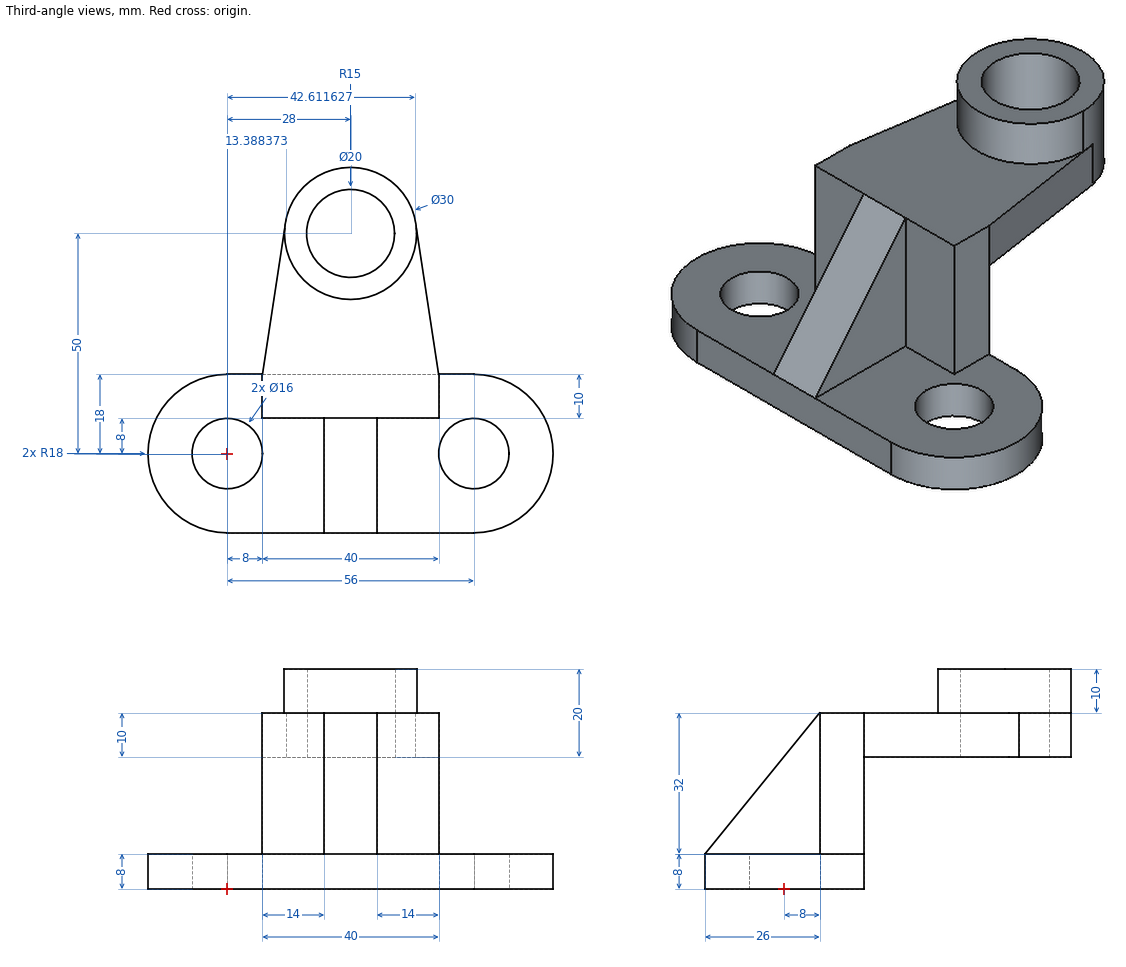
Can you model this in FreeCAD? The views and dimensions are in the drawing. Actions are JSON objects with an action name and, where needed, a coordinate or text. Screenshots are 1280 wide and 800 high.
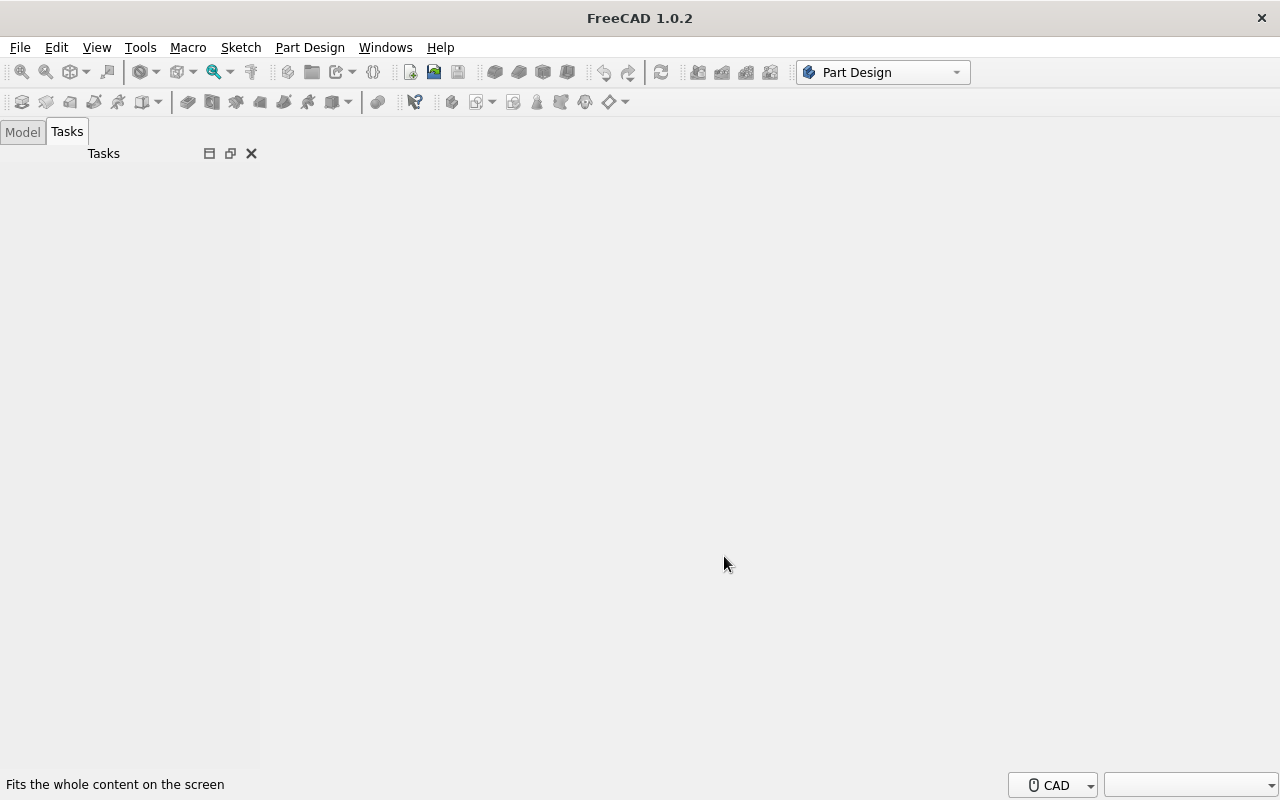
{"action": "left_click", "coordinate": [410, 72]}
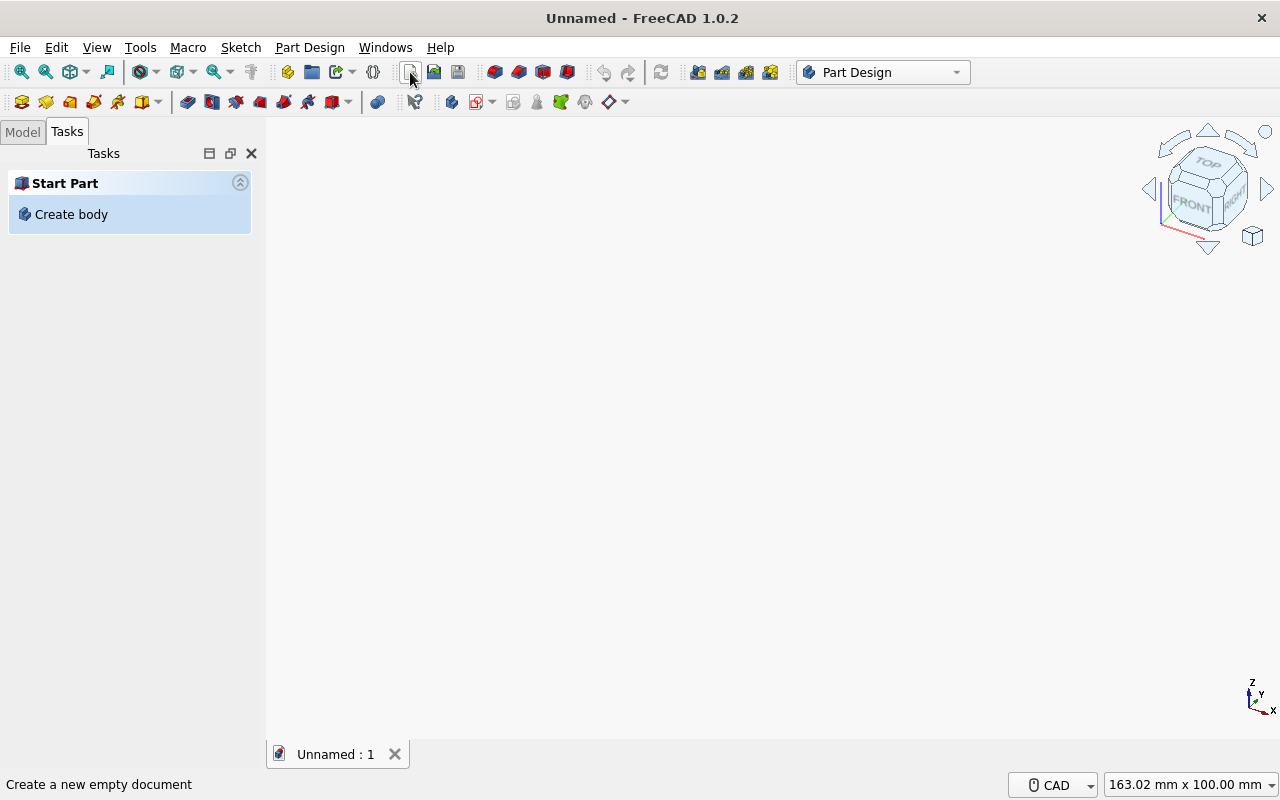
{"action": "left_click", "coordinate": [476, 102]}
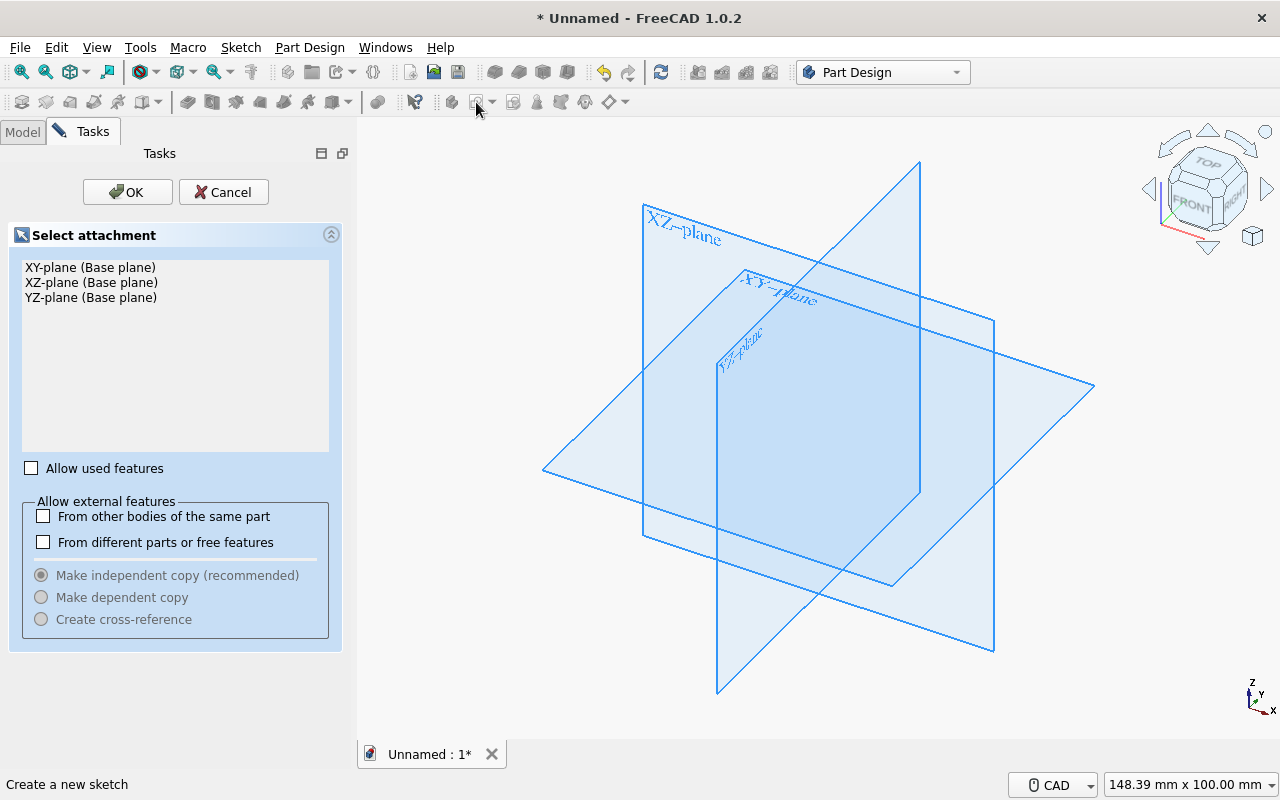
{"action": "left_click", "coordinate": [82, 268]}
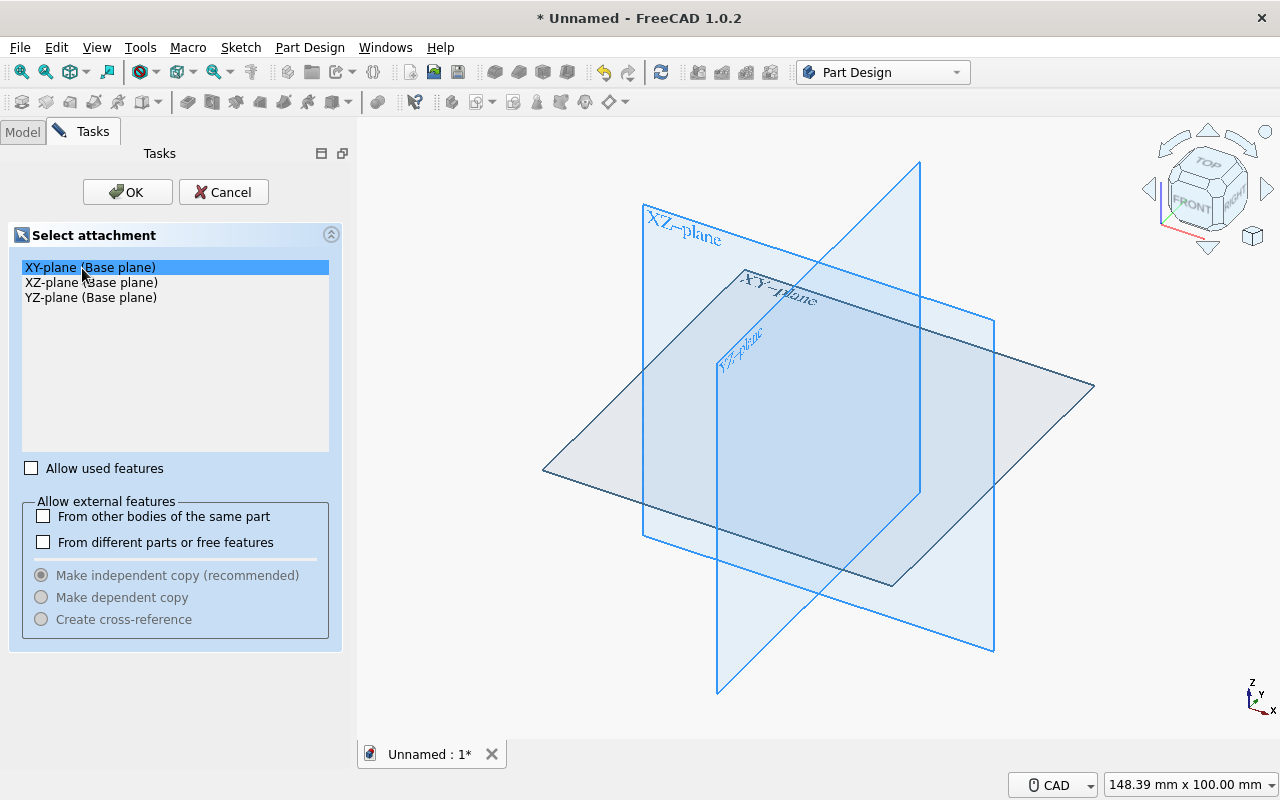
{"action": "left_click", "coordinate": [128, 192]}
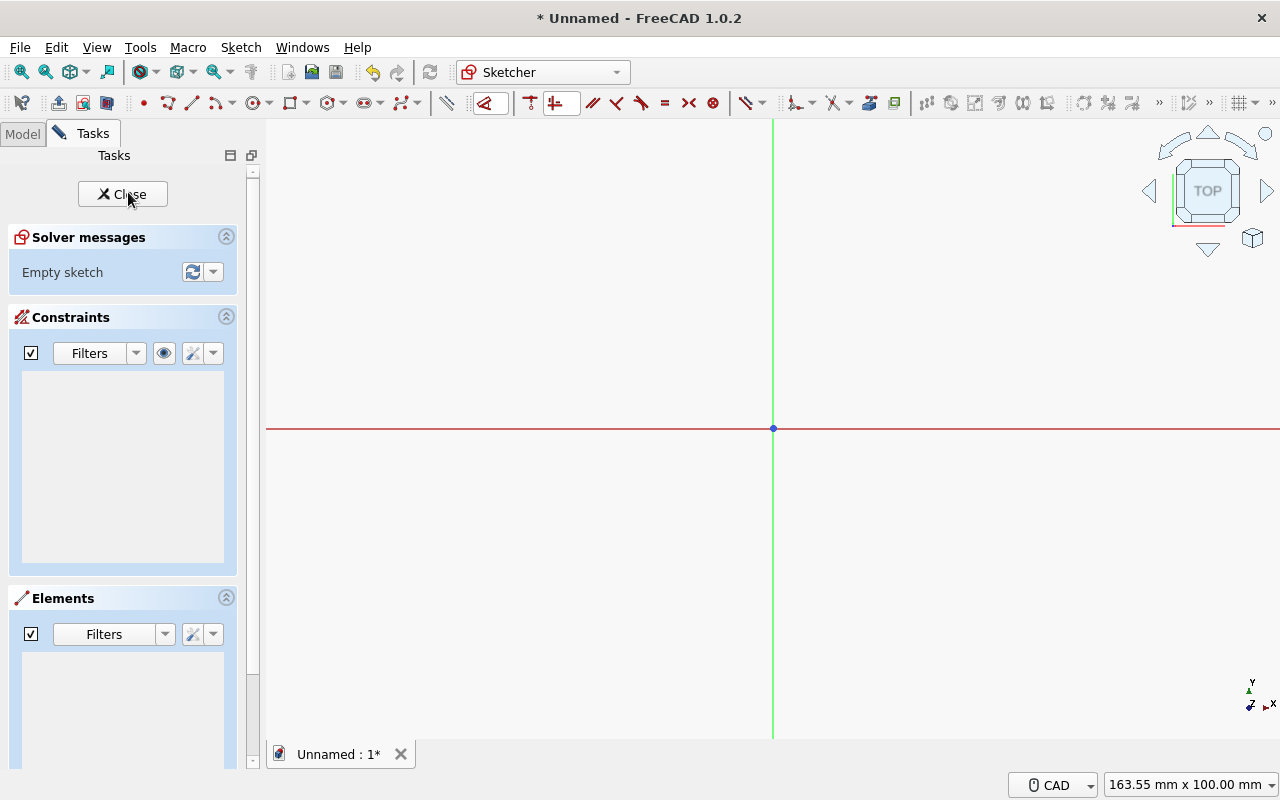
{"action": "scroll", "coordinate": [294, 429], "scroll_direction": "down", "scroll_amount": 1}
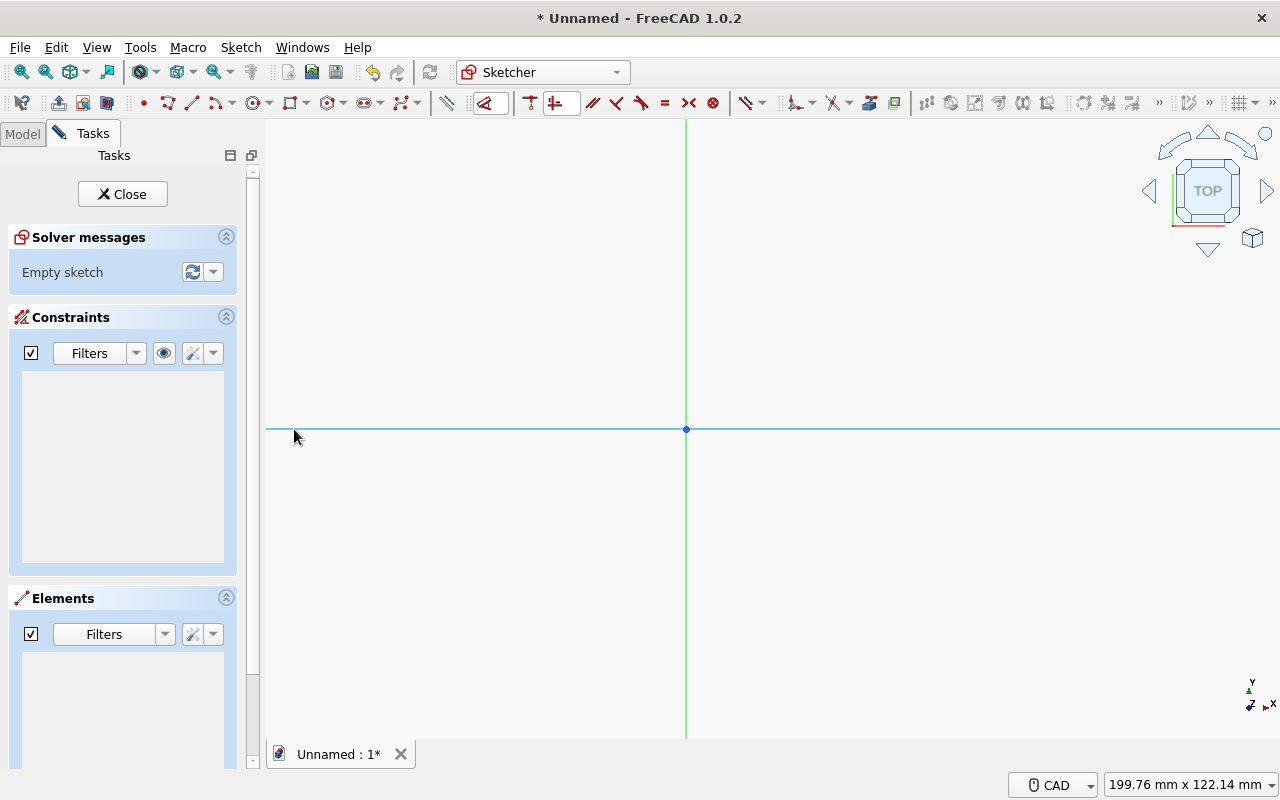
{"action": "left_click", "coordinate": [364, 104]}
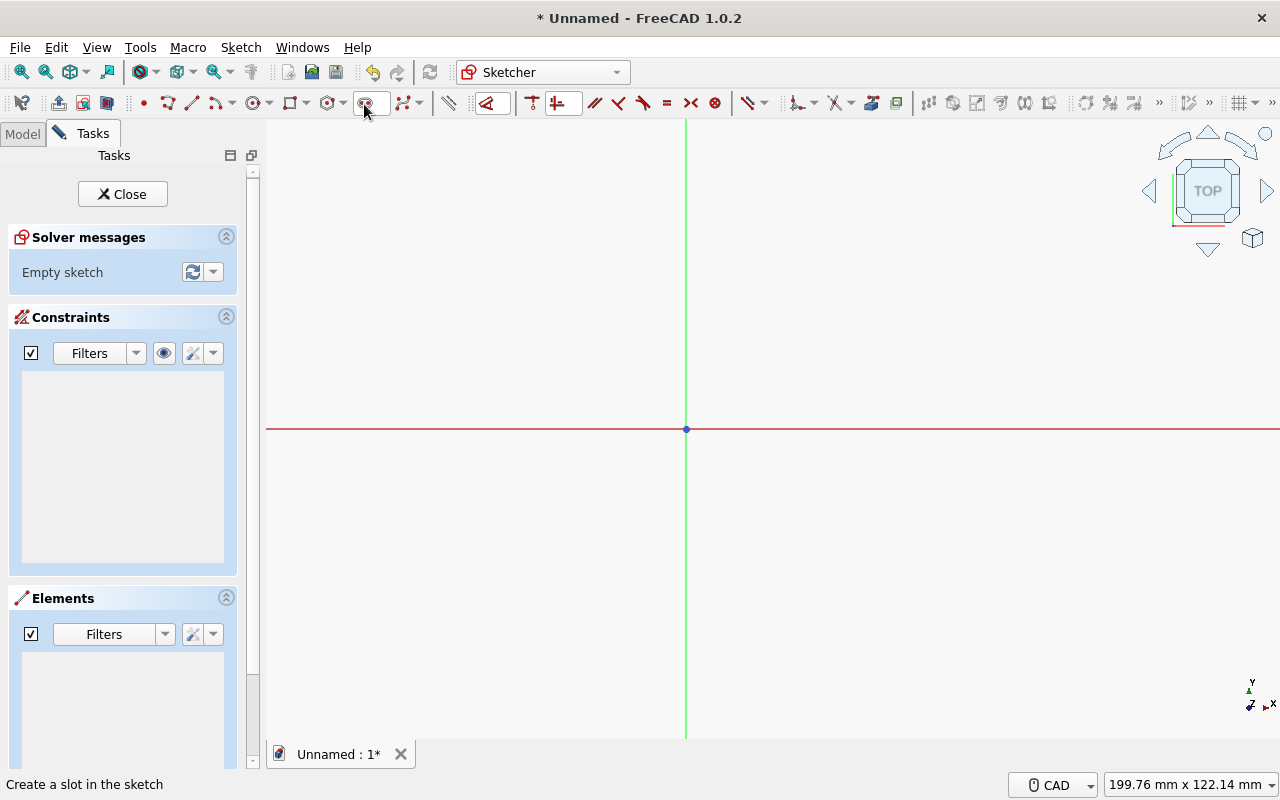
{"action": "left_click", "coordinate": [686, 429]}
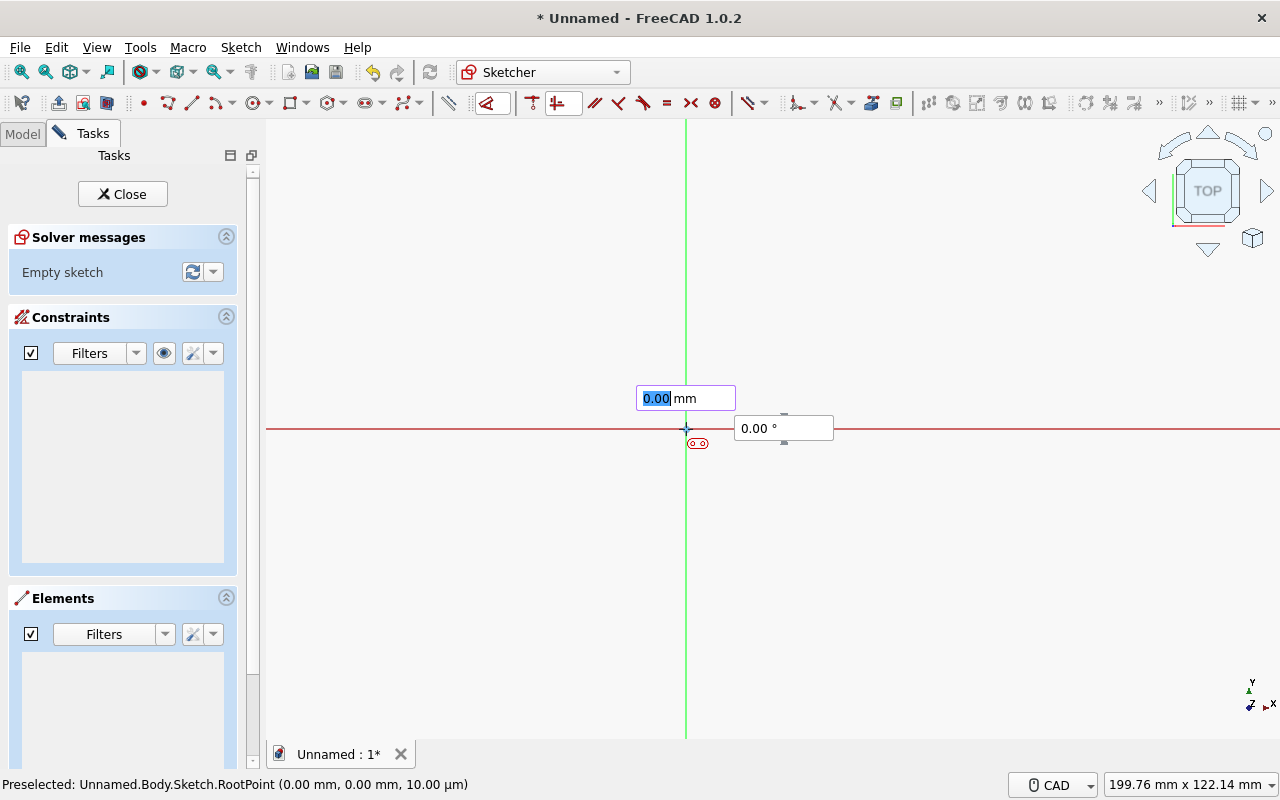
{"action": "left_click", "coordinate": [970, 420]}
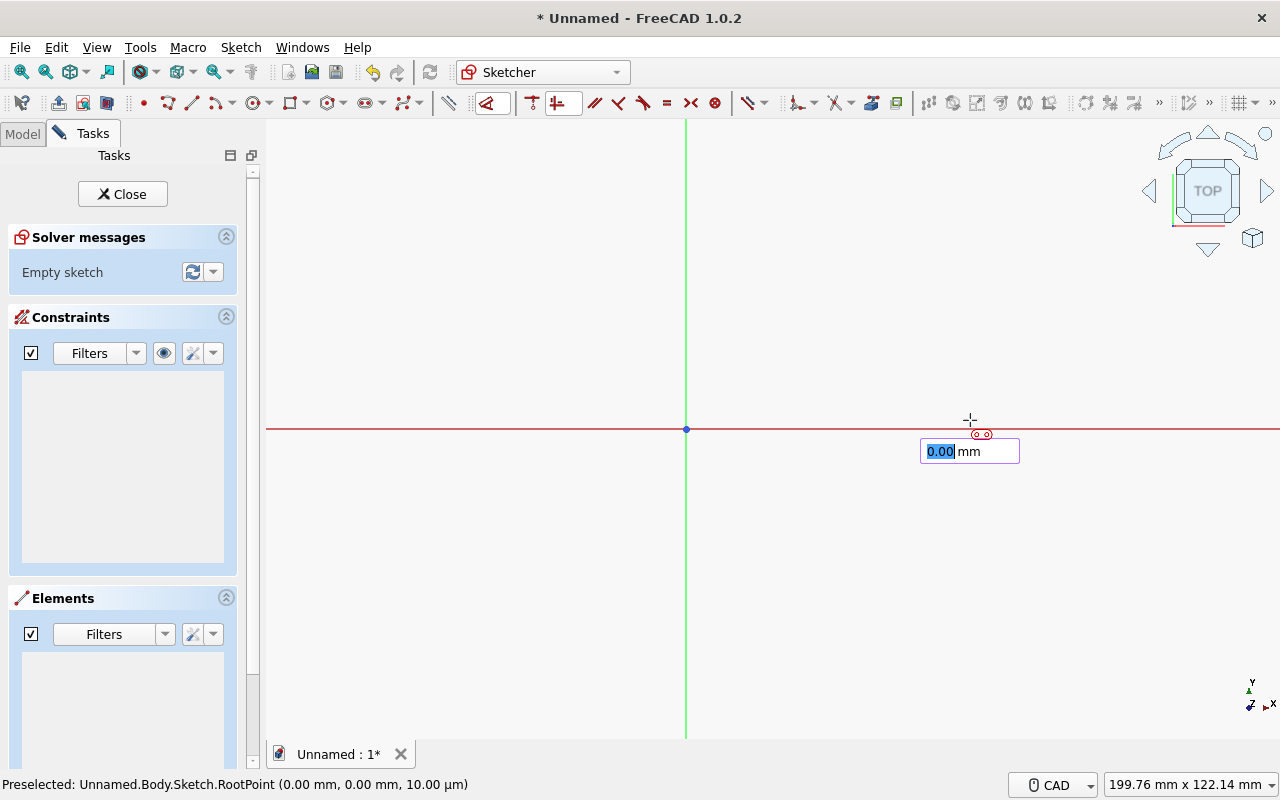
{"action": "left_click", "coordinate": [828, 338]}
{"action": "key", "text": "Escape"}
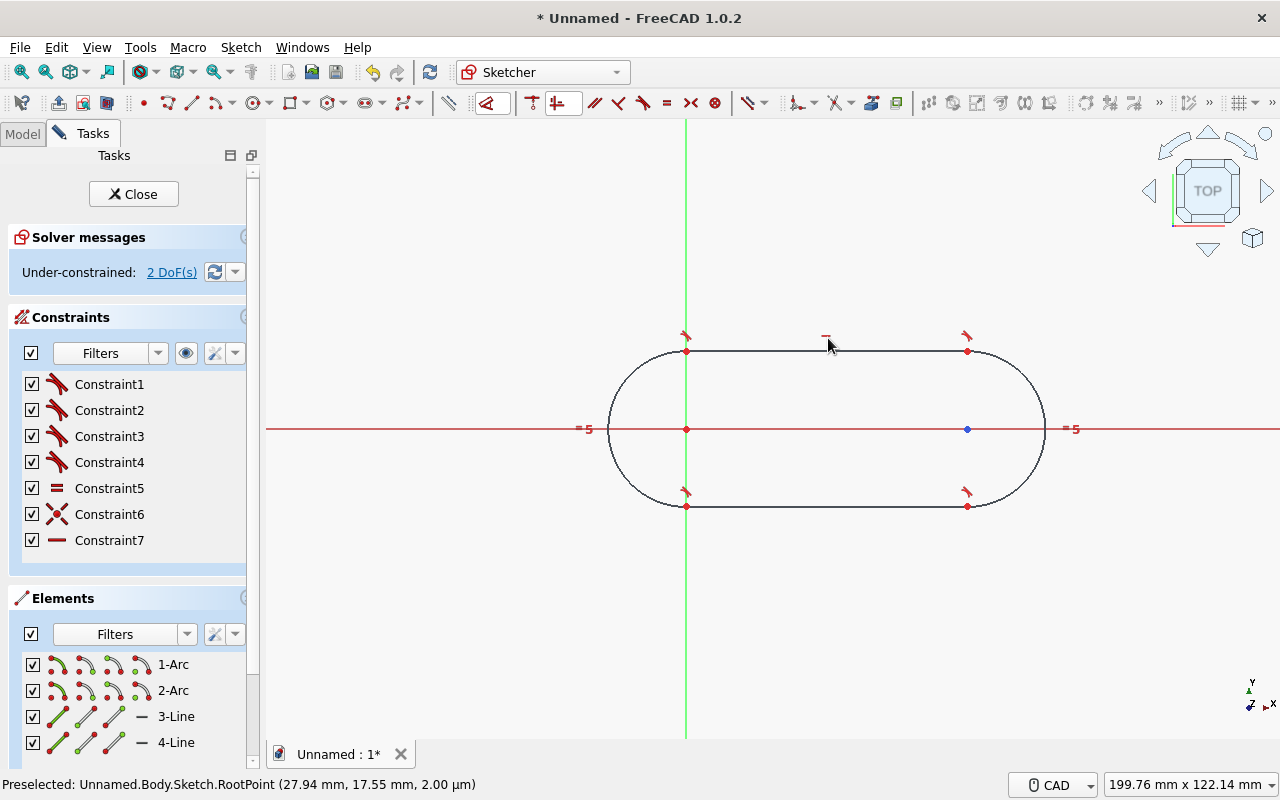
{"action": "left_click", "coordinate": [623, 383]}